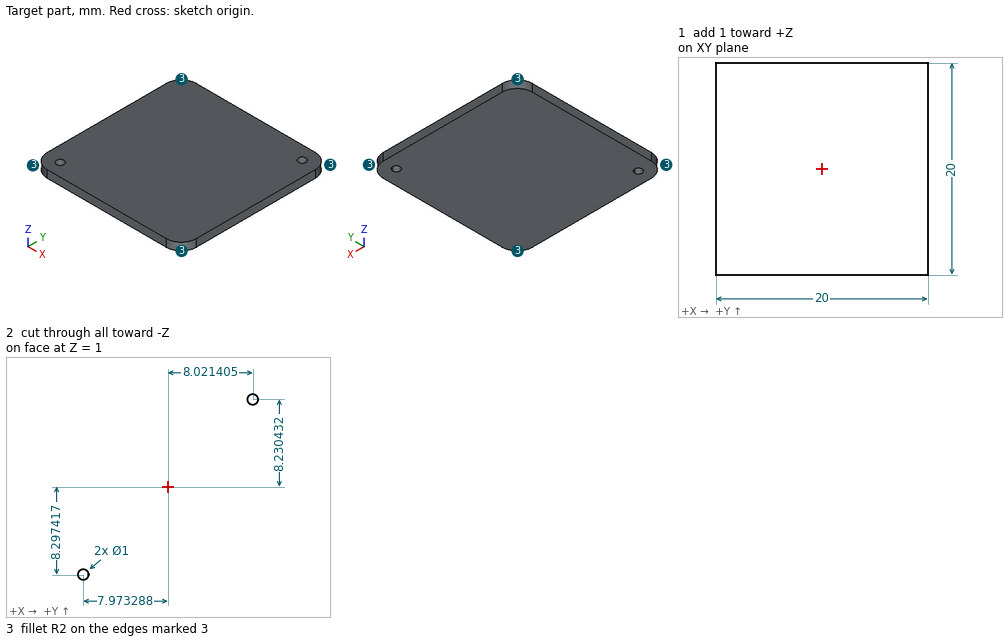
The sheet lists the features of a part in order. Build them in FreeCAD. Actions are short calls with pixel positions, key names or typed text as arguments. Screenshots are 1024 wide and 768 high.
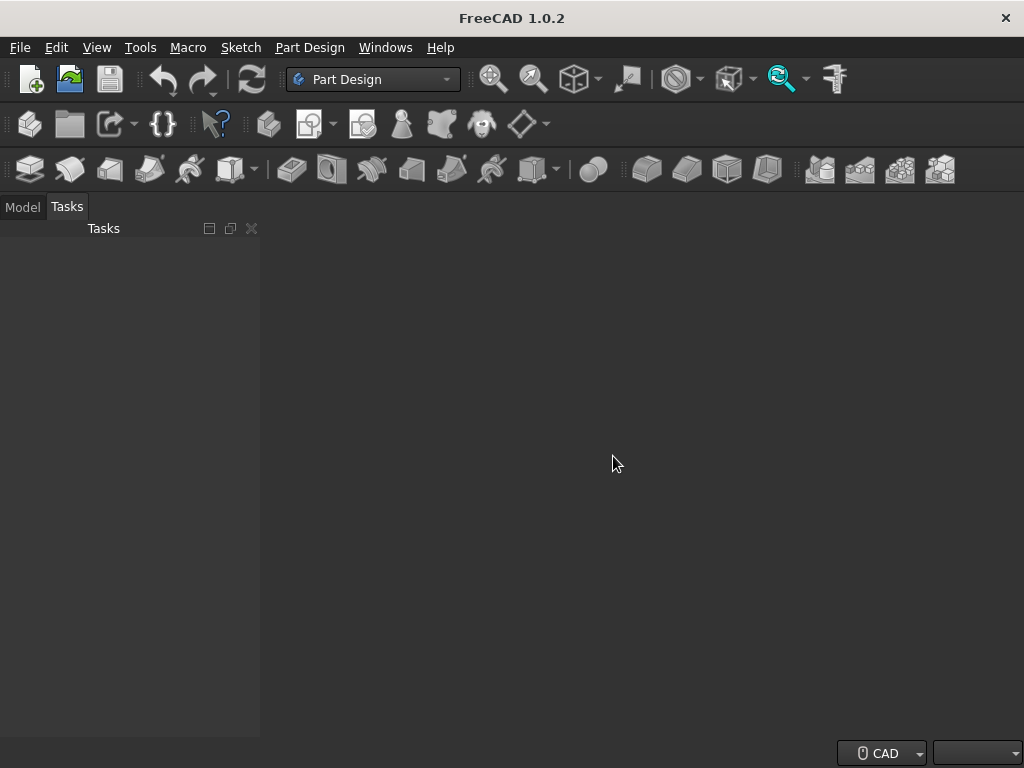
key(ctrl+n)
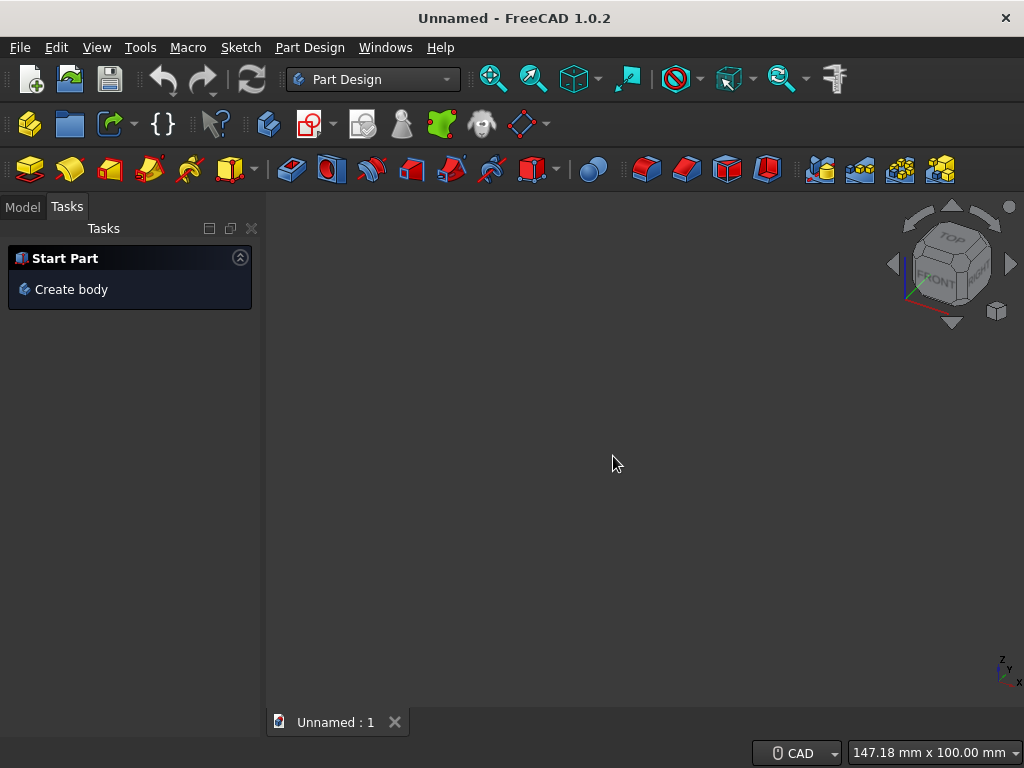
click(310, 124)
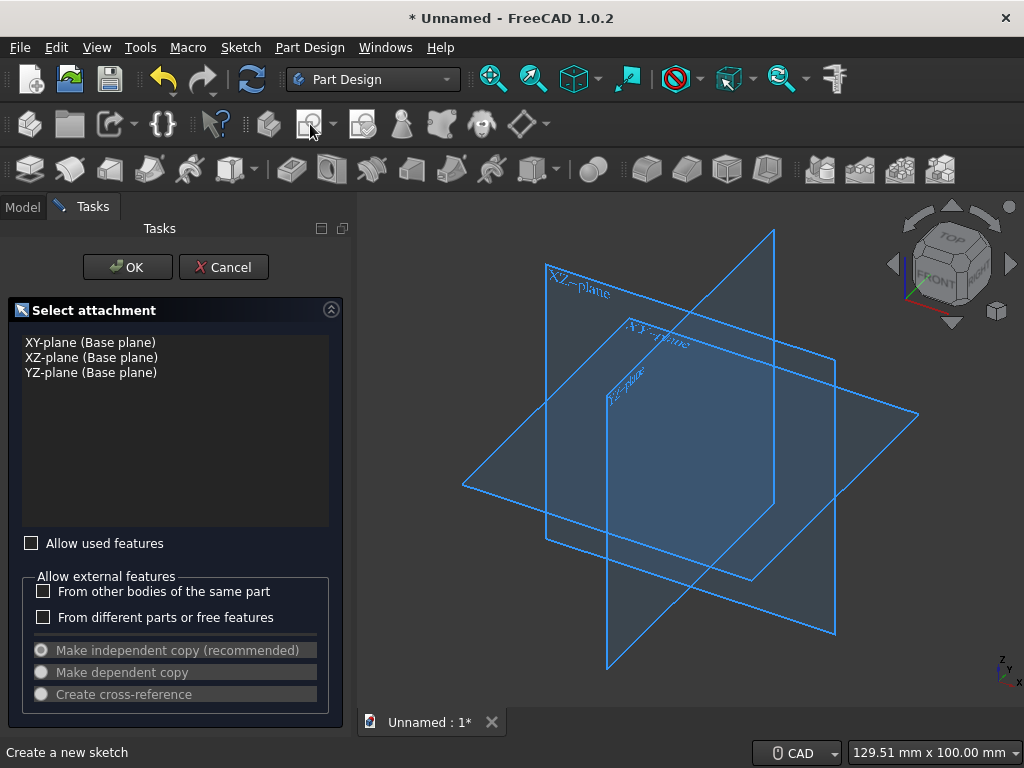
click(82, 342)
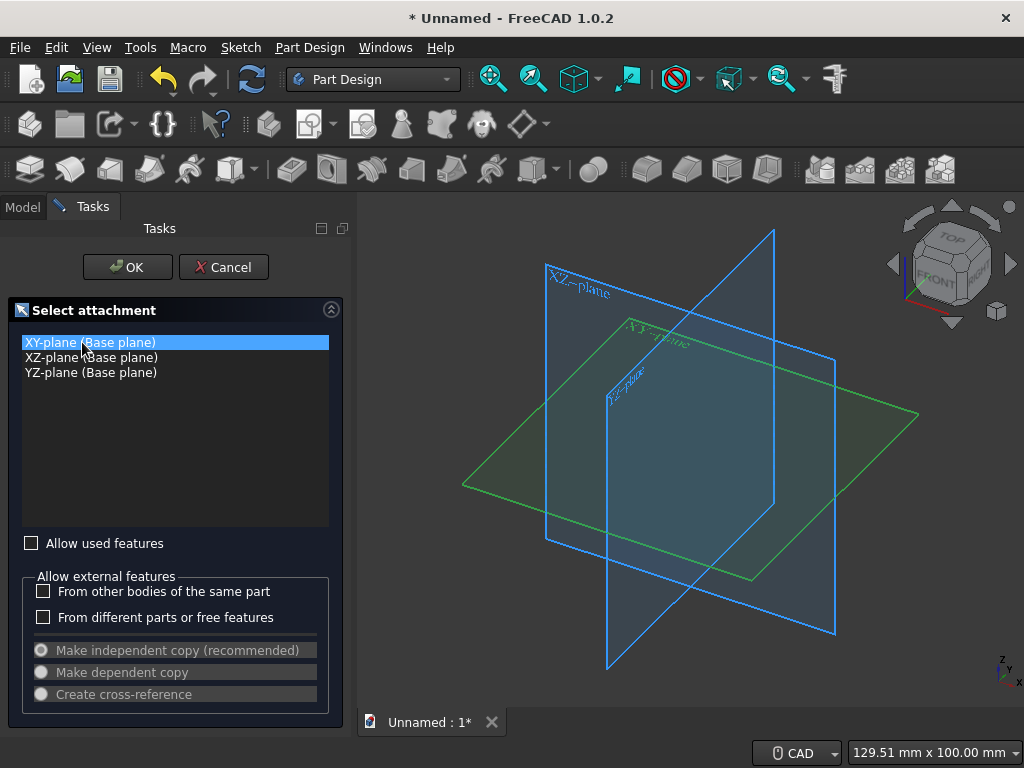
click(128, 267)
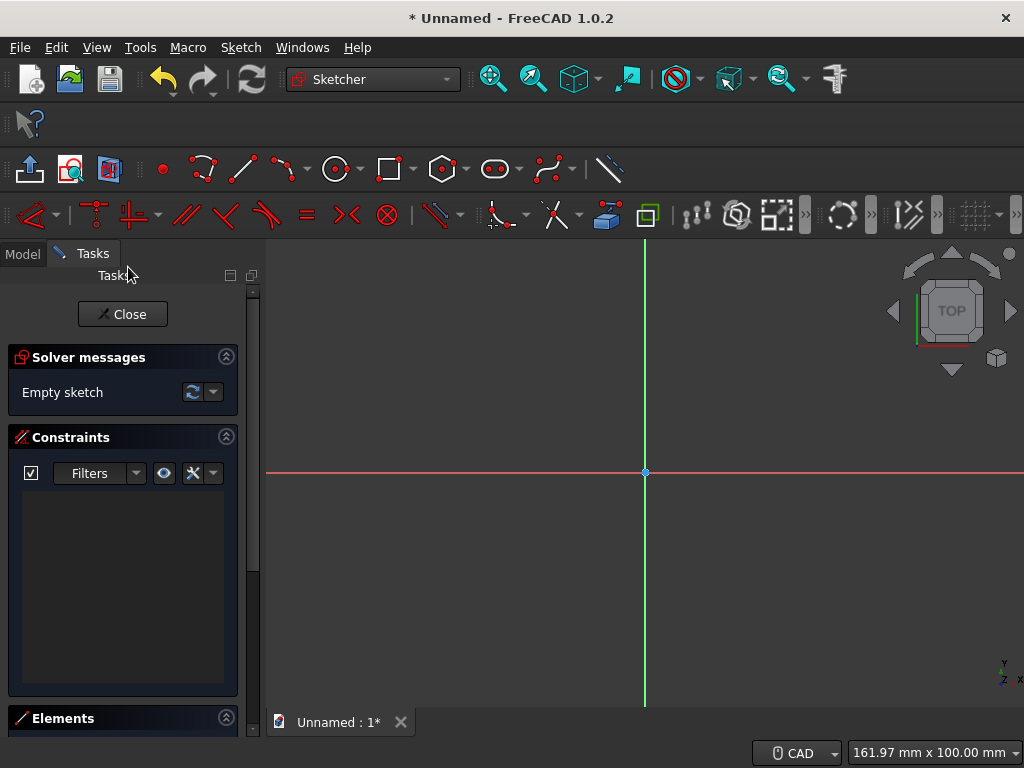
scroll(675, 473, up, 6)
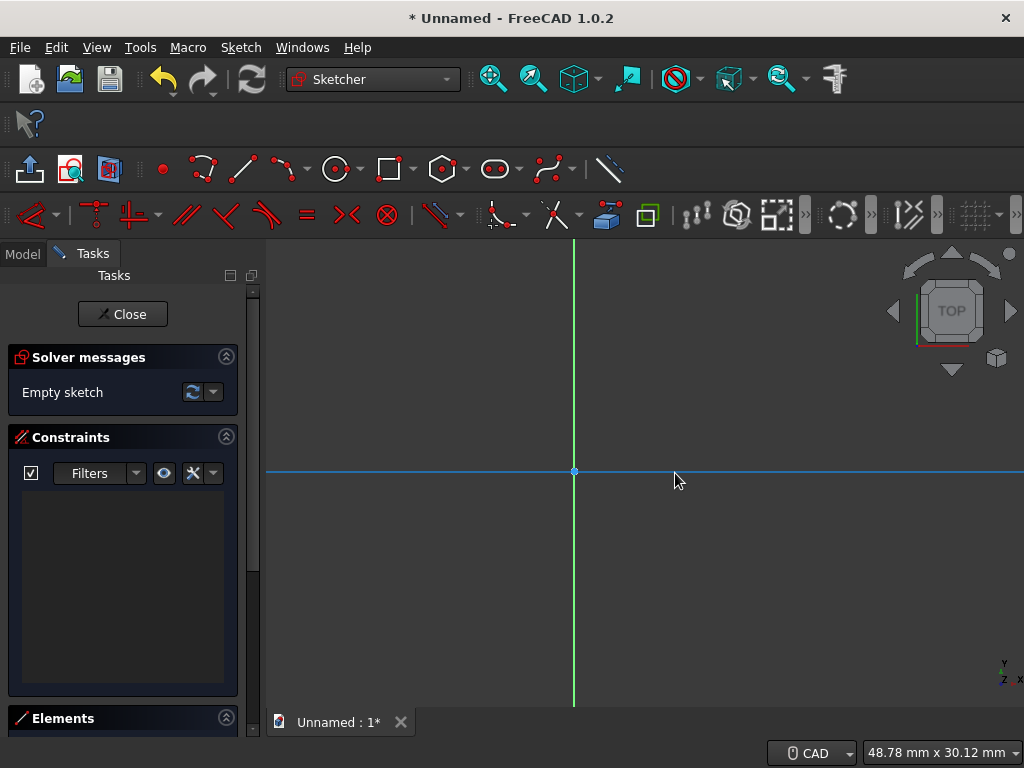
key(g)
key(v)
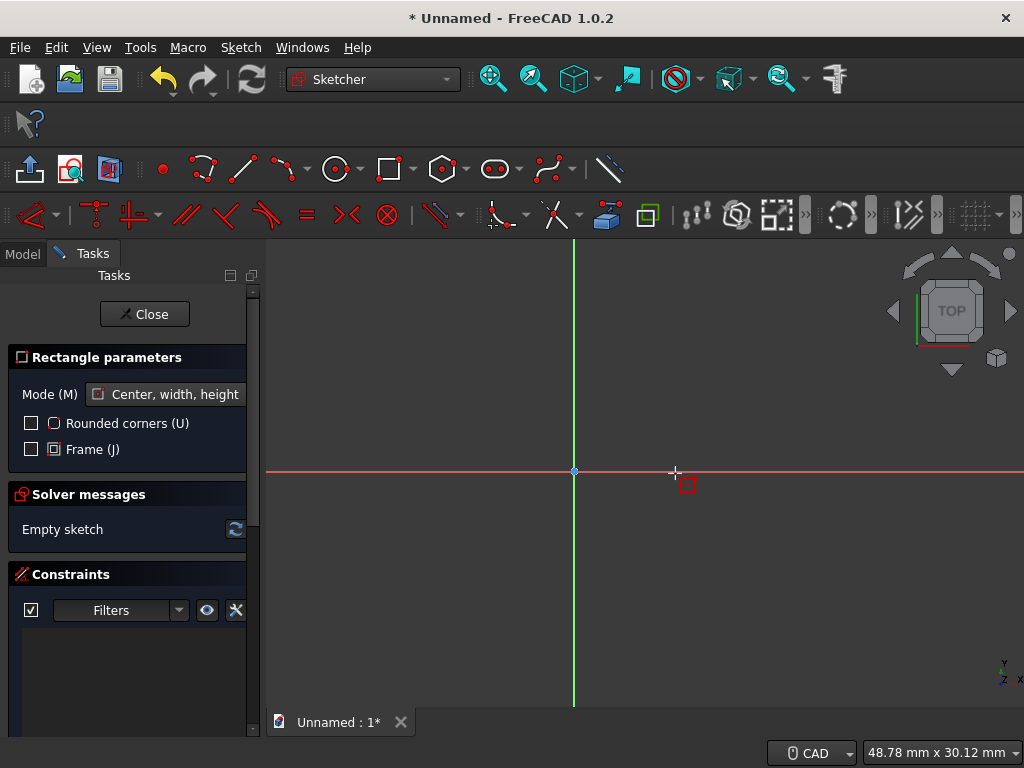
click(574, 472)
move(730, 316)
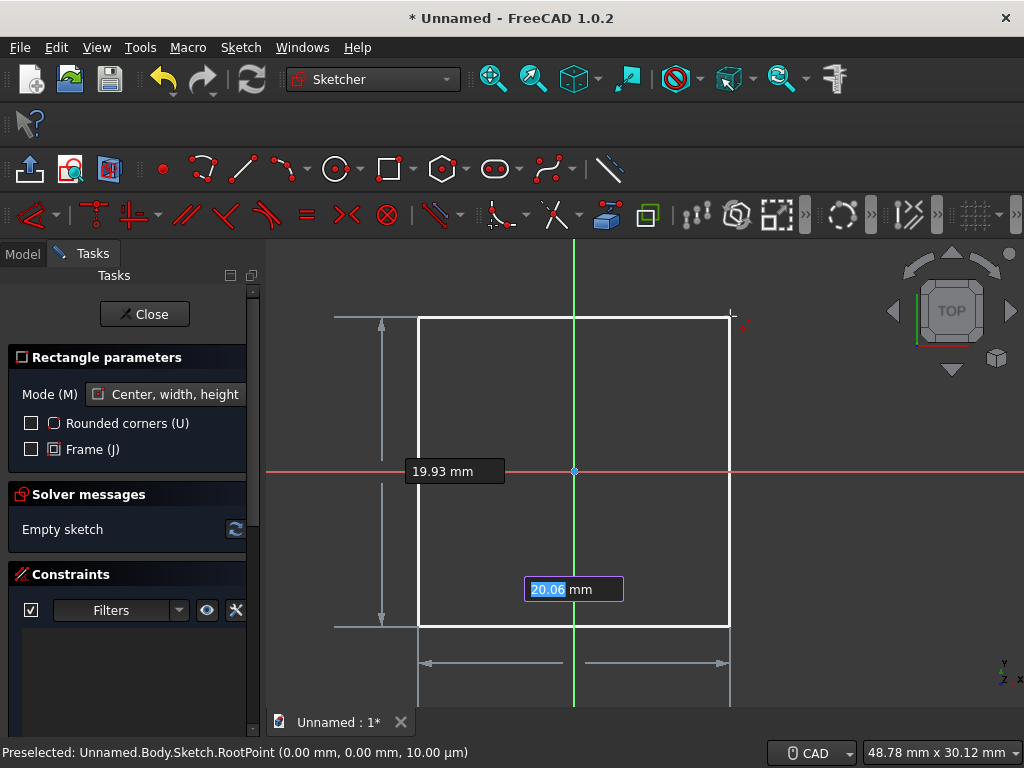
text(20)
key(Tab)
text(20)
key(Return)
key(Escape)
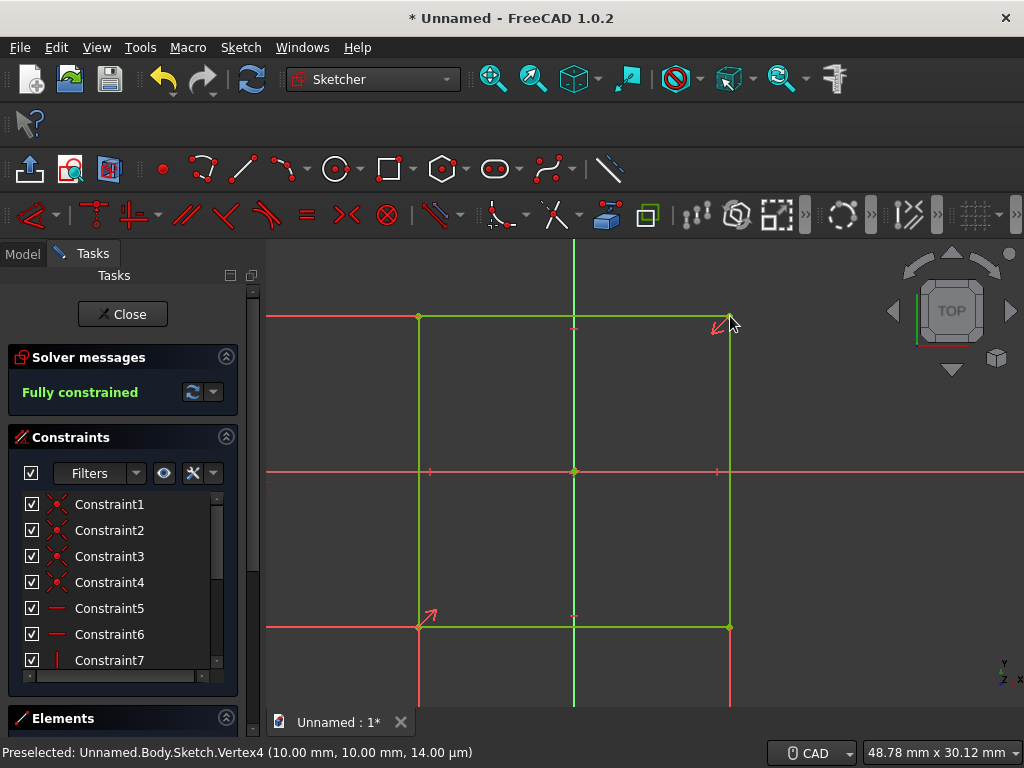
click(123, 314)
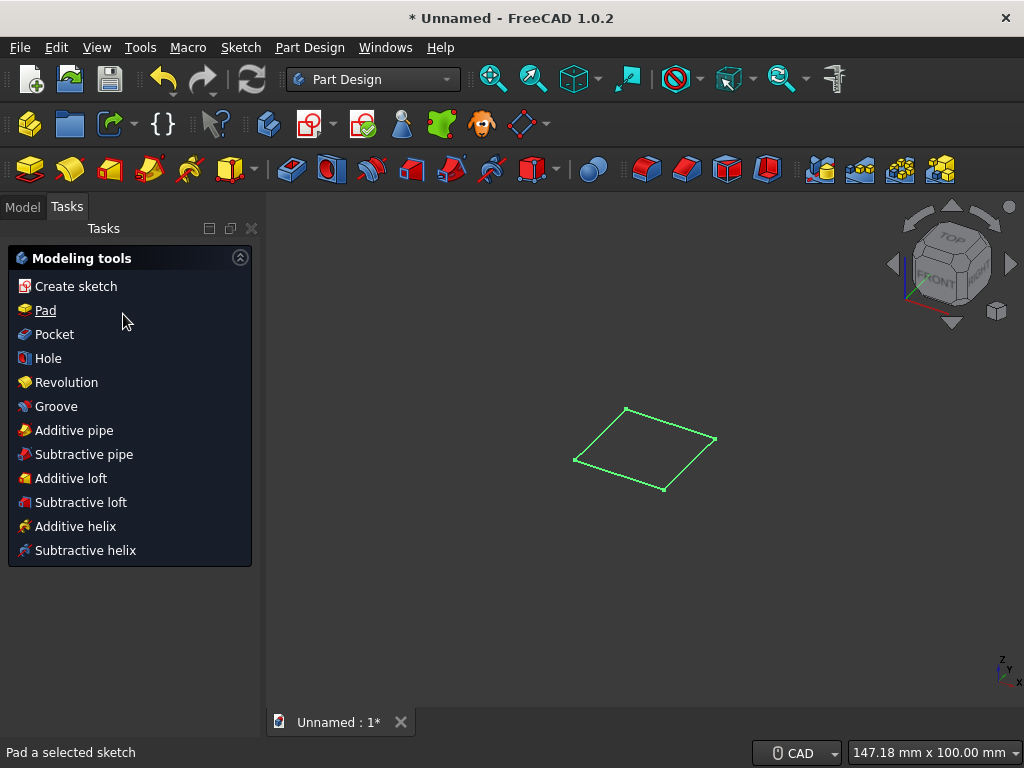
click(30, 170)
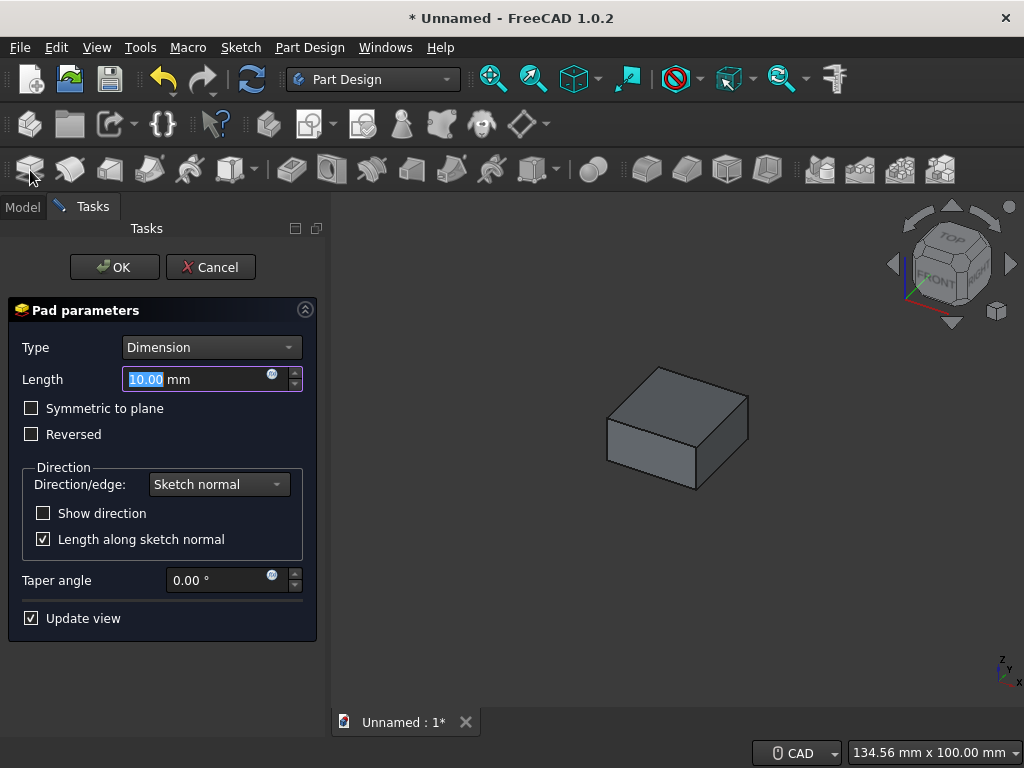
text(1)
key(Tab)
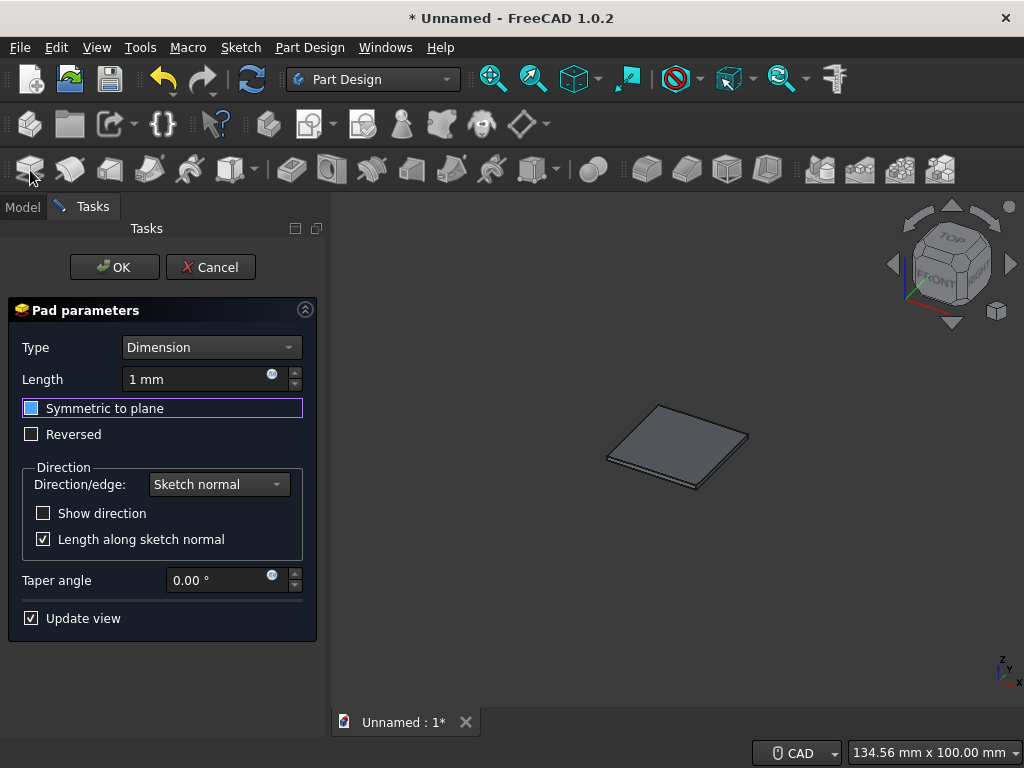
click(115, 267)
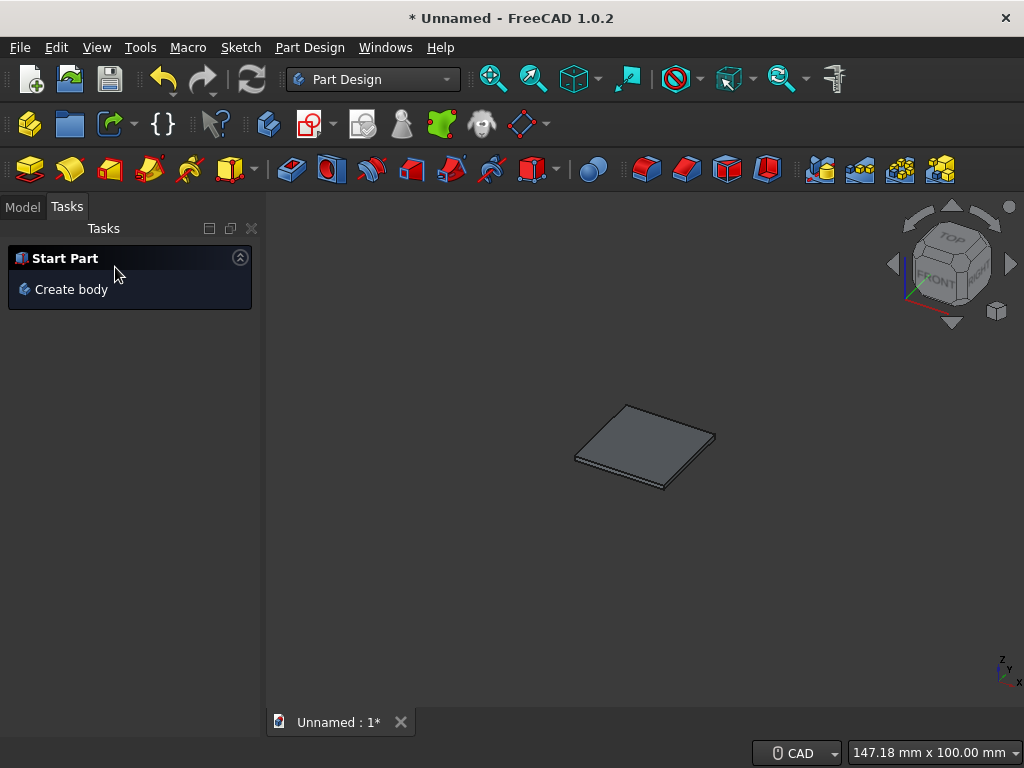
key(v)
key(f)